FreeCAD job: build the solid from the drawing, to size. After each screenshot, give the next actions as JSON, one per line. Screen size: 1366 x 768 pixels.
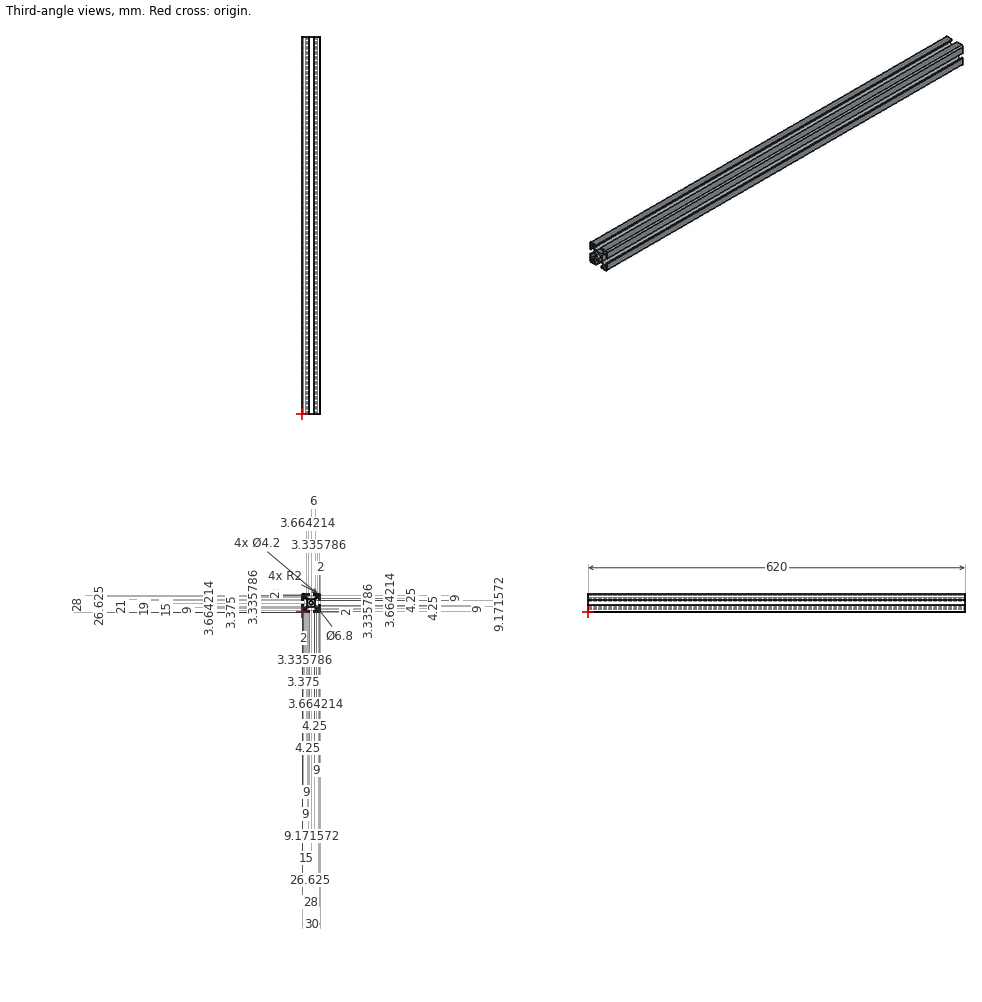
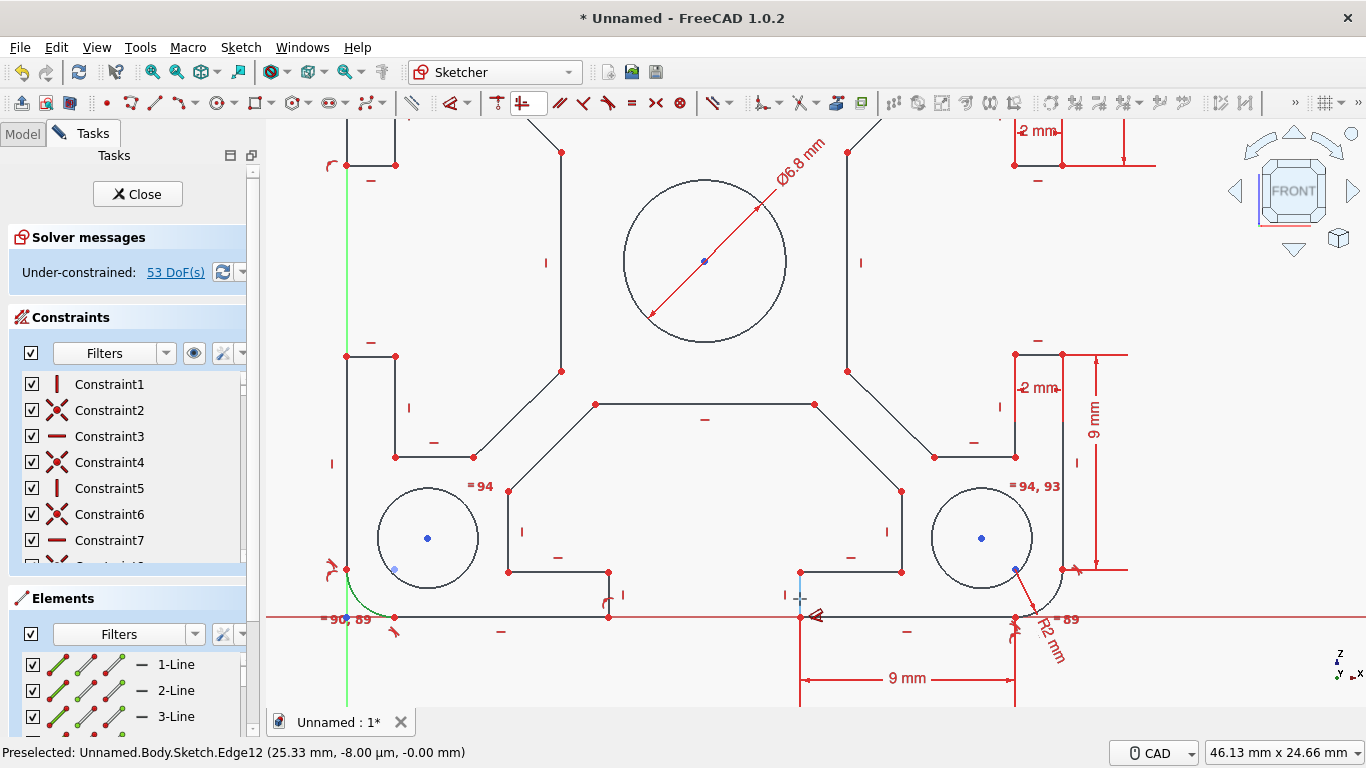
{"action": "left_click", "coordinate": [800, 599]}
{"action": "left_click", "coordinate": [834, 595]}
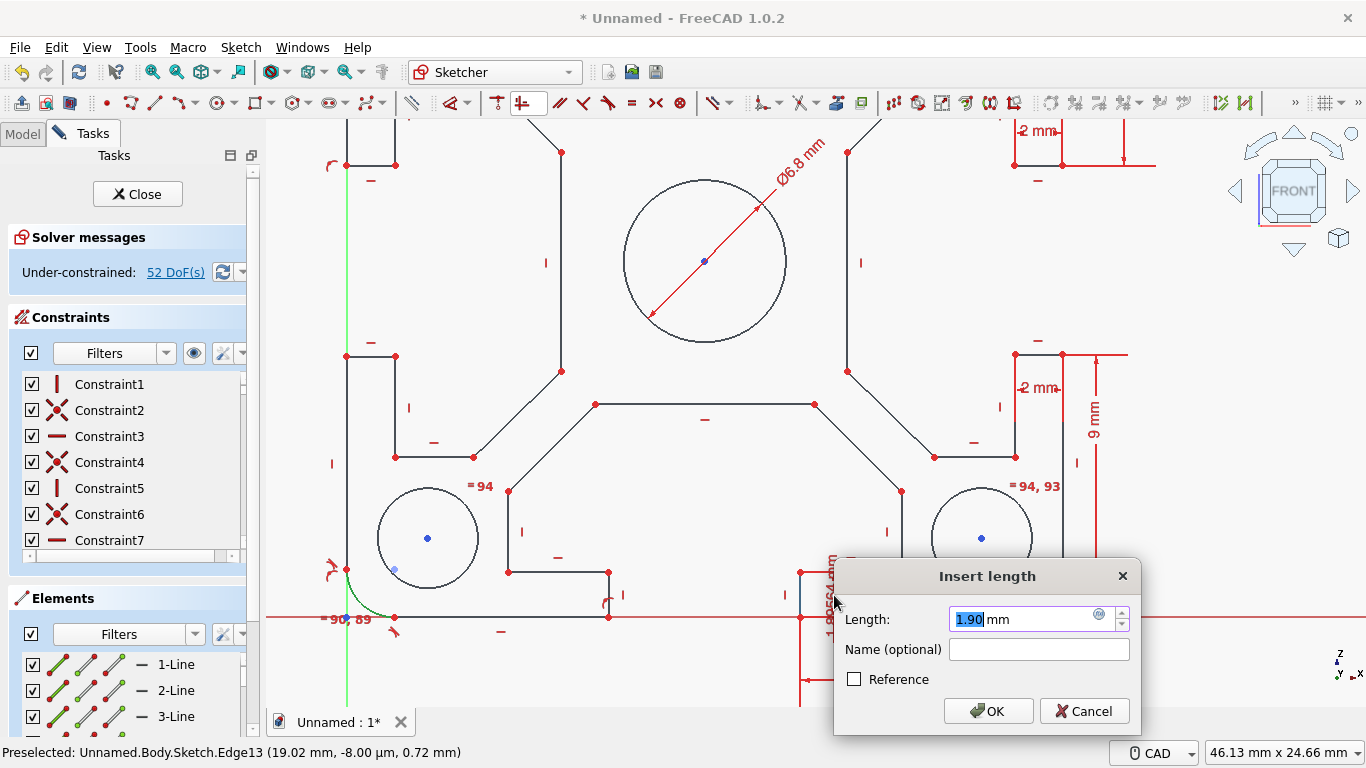
{"action": "type", "text": "2"}
{"action": "key", "text": "Return"}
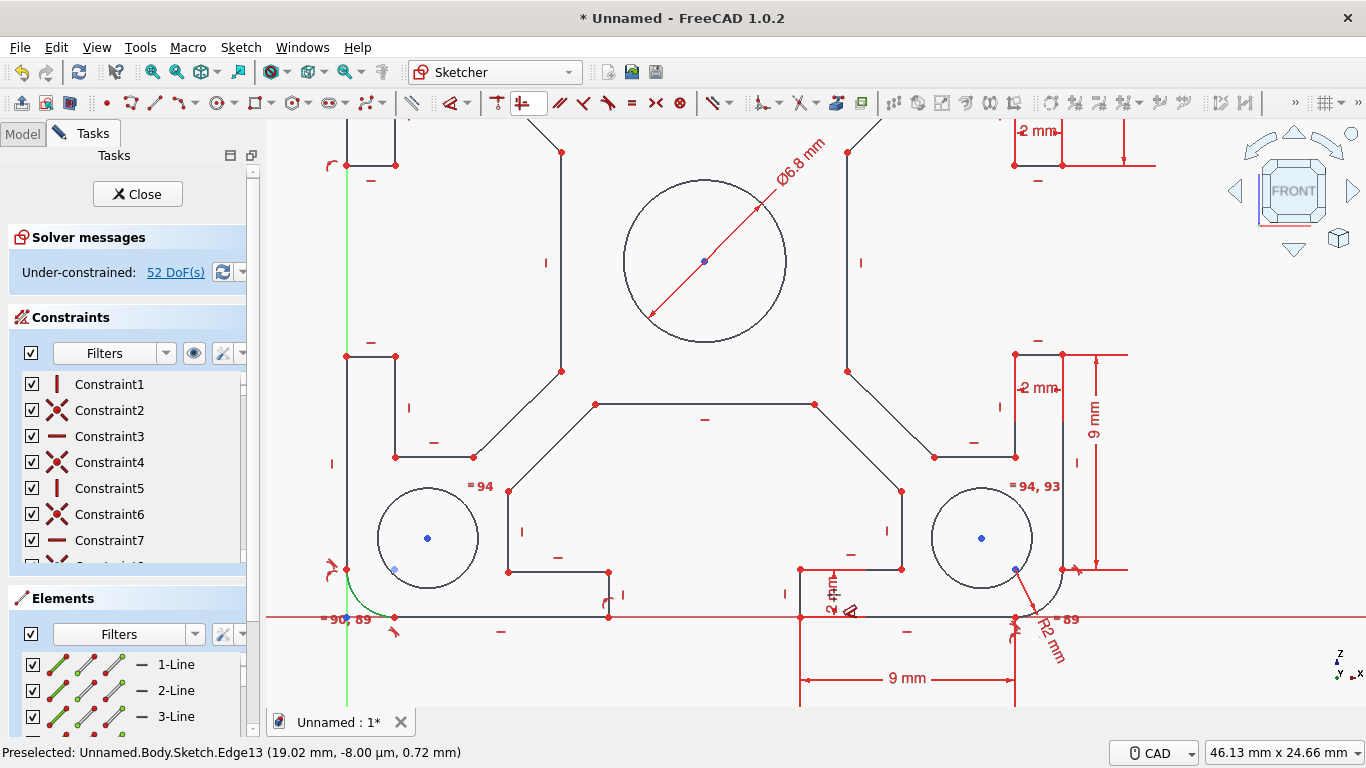
{"action": "left_click", "coordinate": [609, 586]}
{"action": "left_click", "coordinate": [575, 595]}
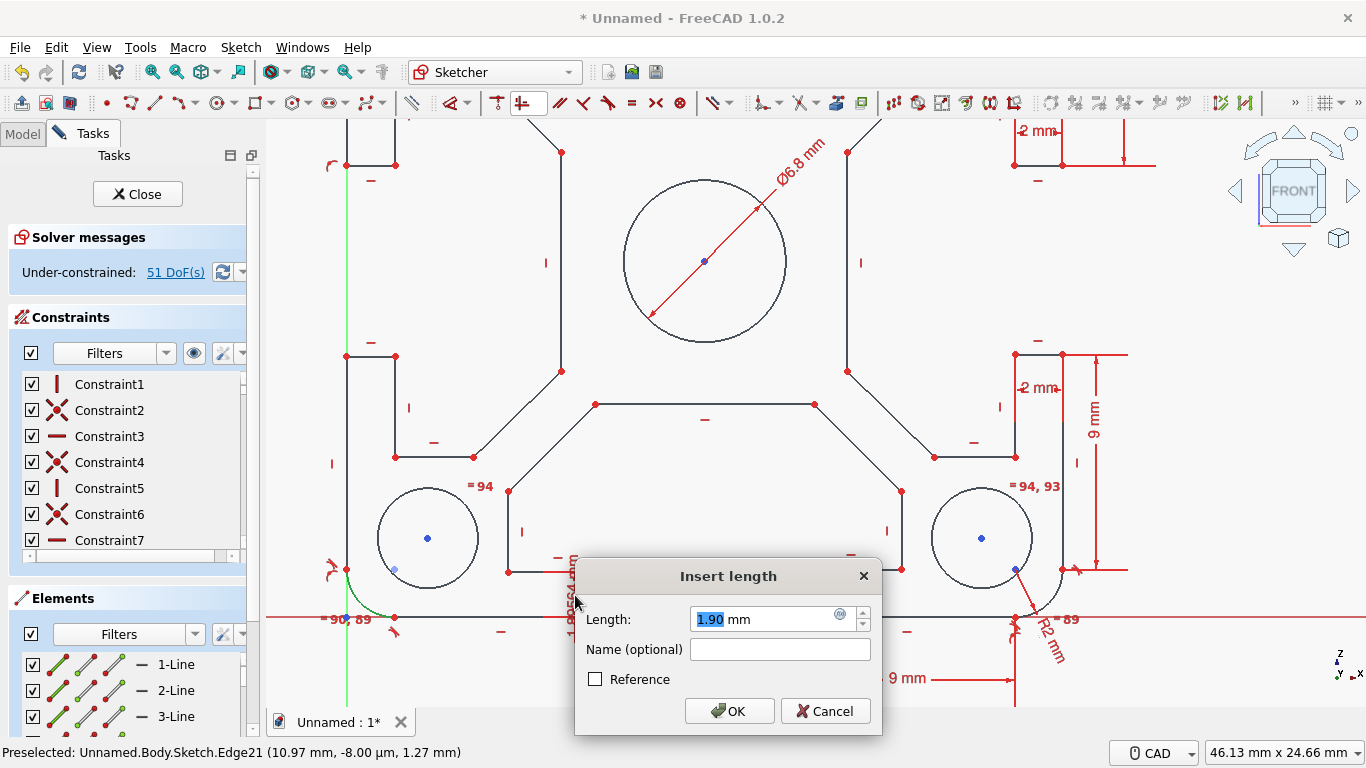
{"action": "type", "text": "2"}
{"action": "key", "text": "Return"}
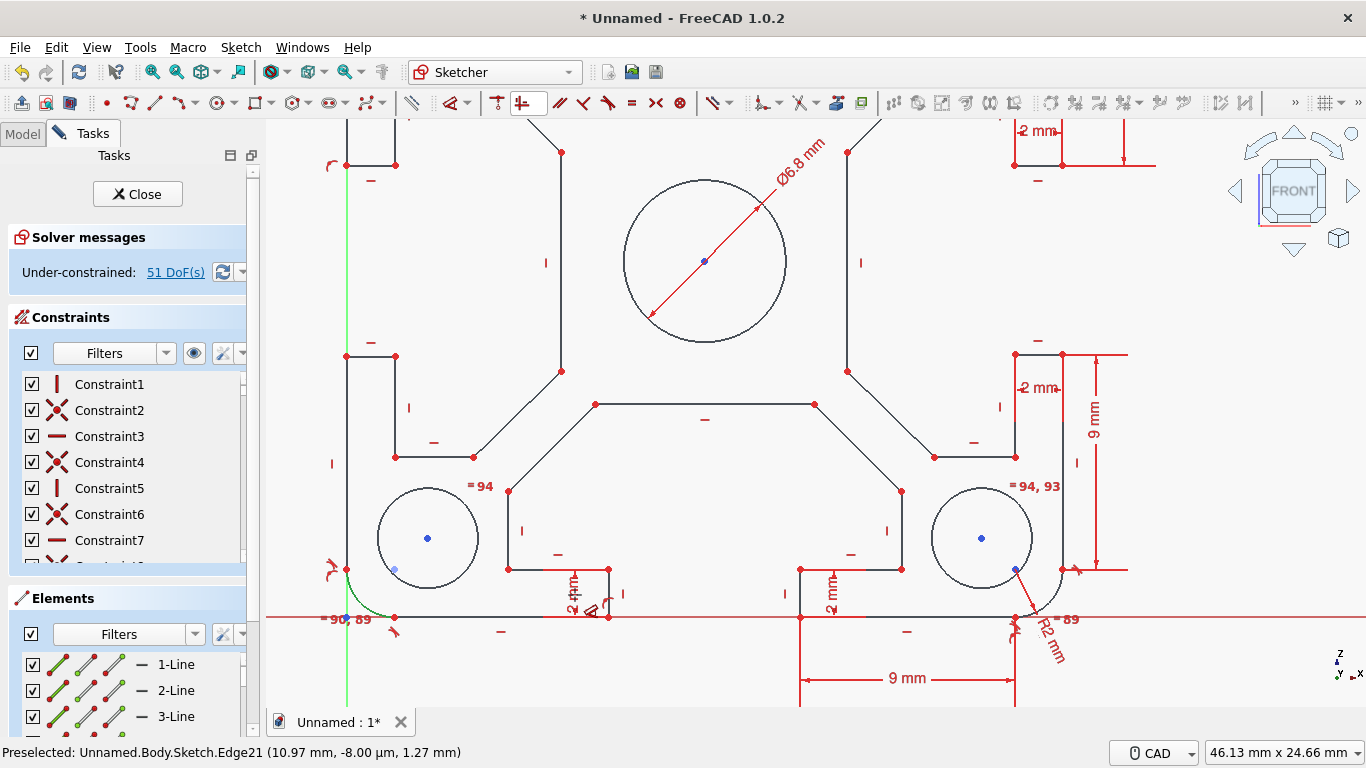
{"action": "left_click", "coordinate": [544, 617]}
{"action": "left_click", "coordinate": [502, 651]}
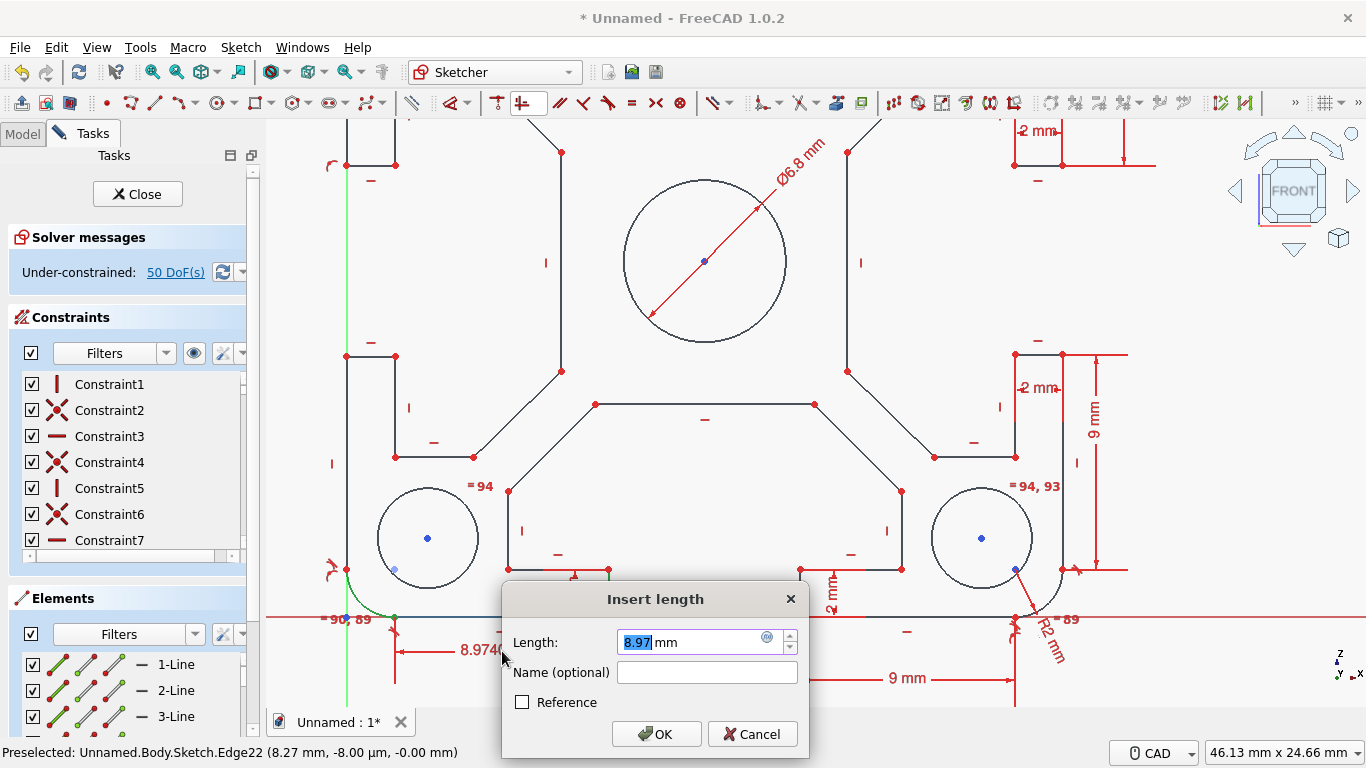
{"action": "type", "text": "9"}
{"action": "key", "text": "Return"}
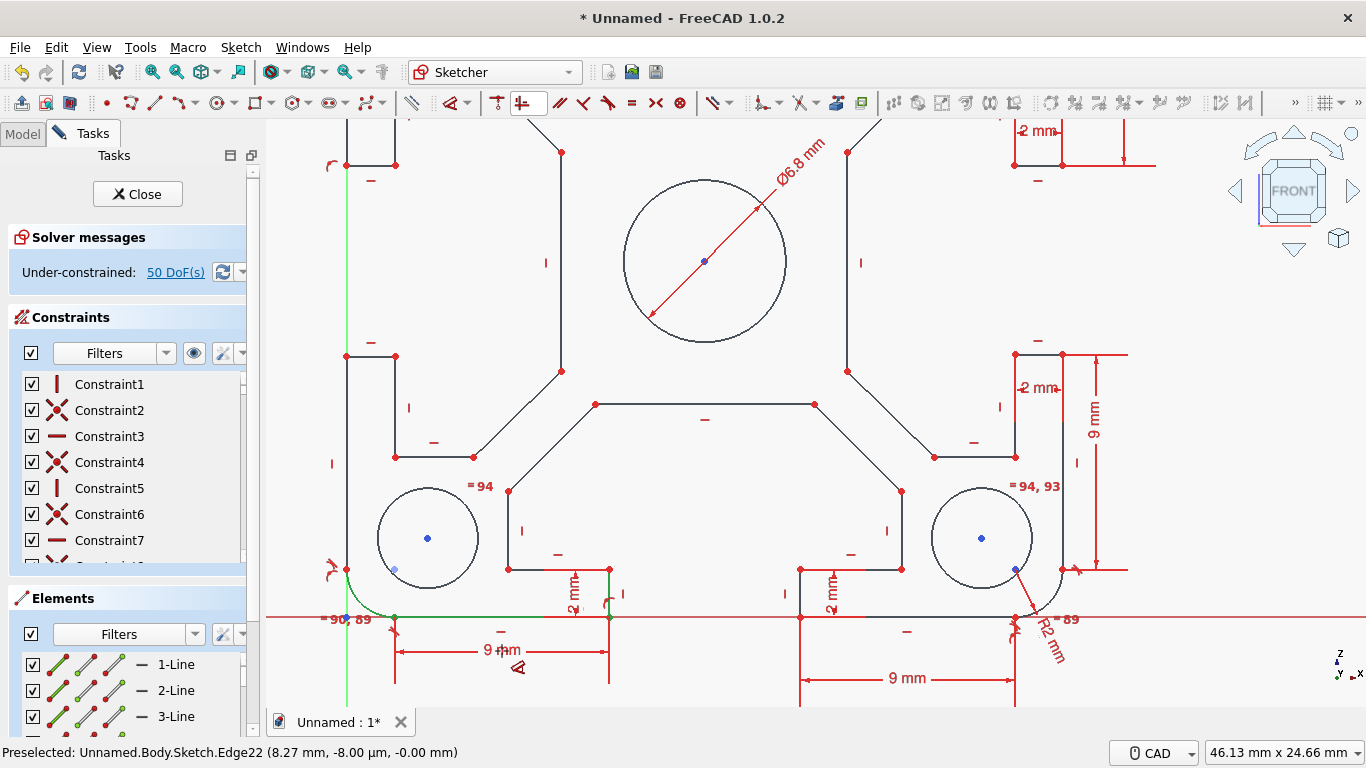
{"action": "left_click", "coordinate": [347, 506]}
{"action": "left_click", "coordinate": [313, 463]}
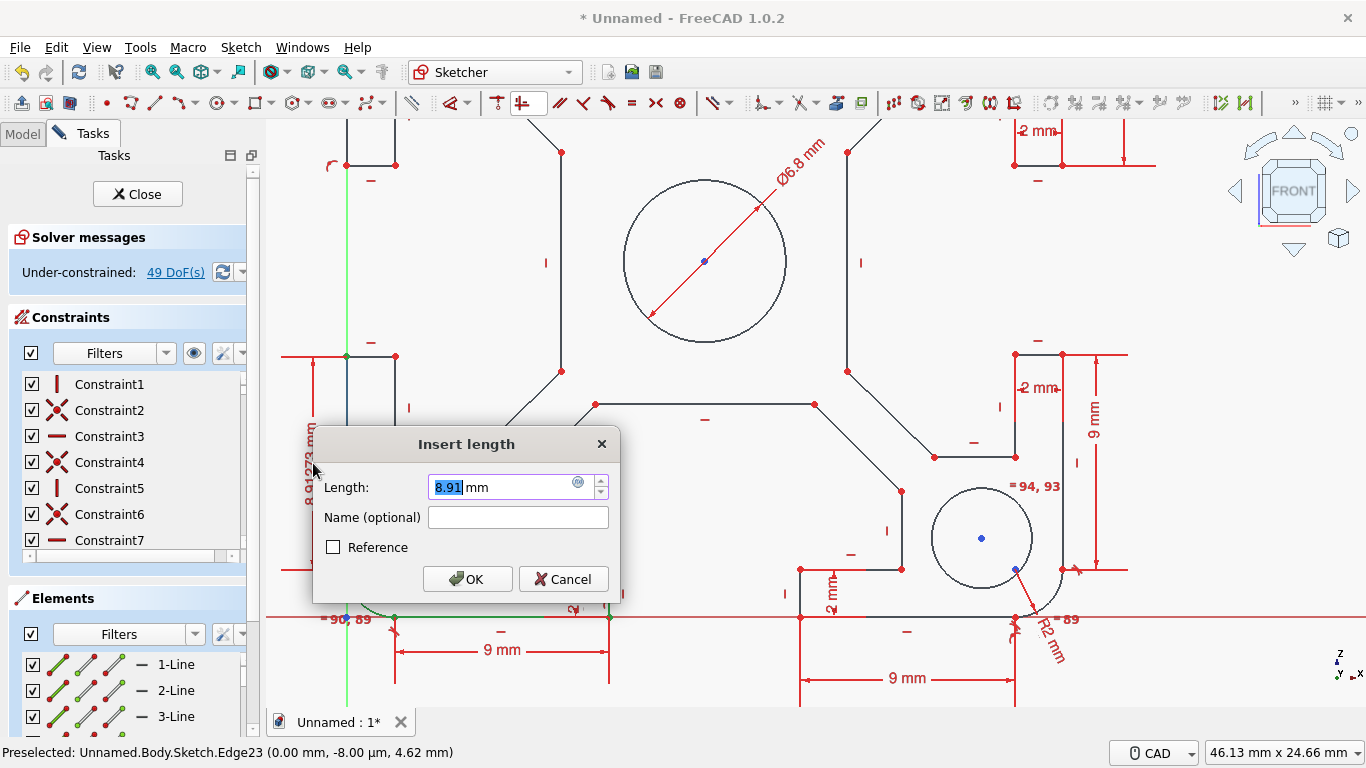
{"action": "type", "text": "9"}
{"action": "key", "text": "Return"}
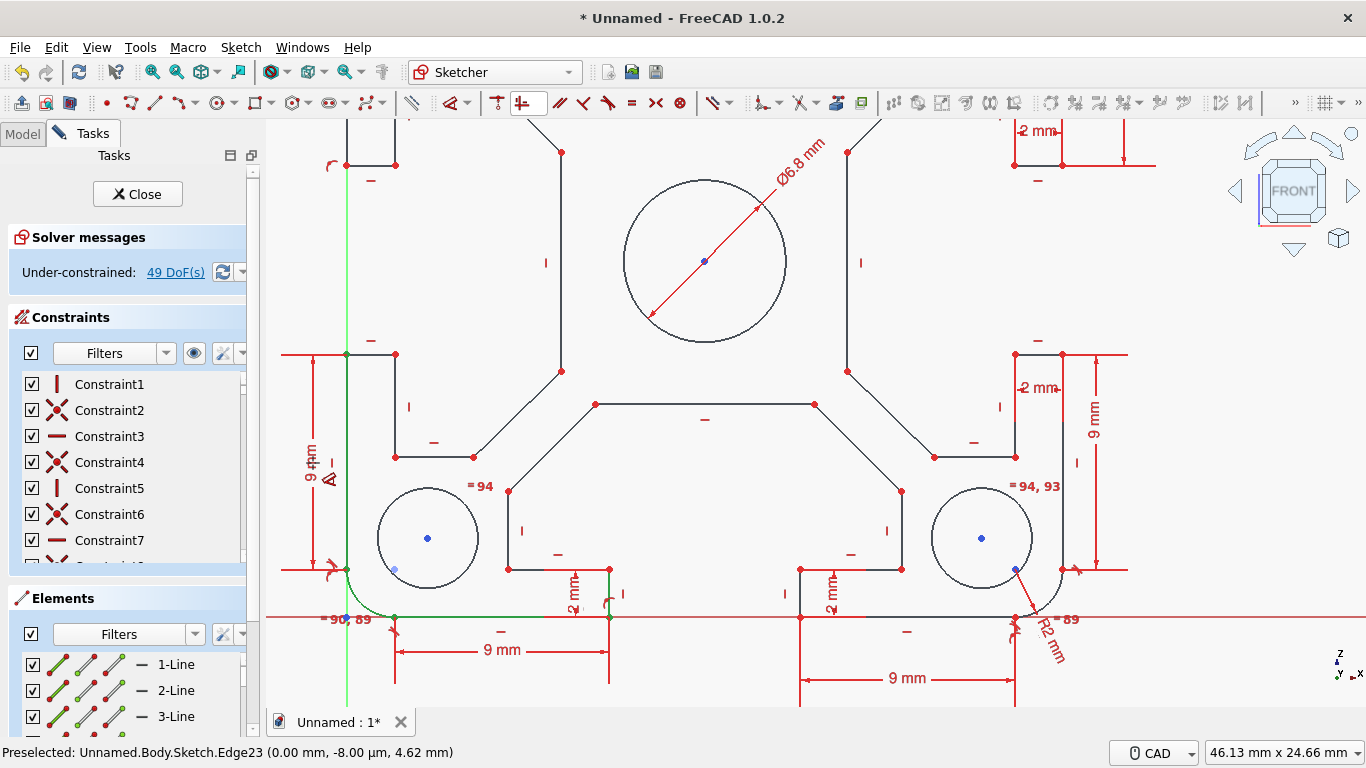
{"action": "left_click", "coordinate": [361, 355]}
{"action": "left_click", "coordinate": [371, 389]}